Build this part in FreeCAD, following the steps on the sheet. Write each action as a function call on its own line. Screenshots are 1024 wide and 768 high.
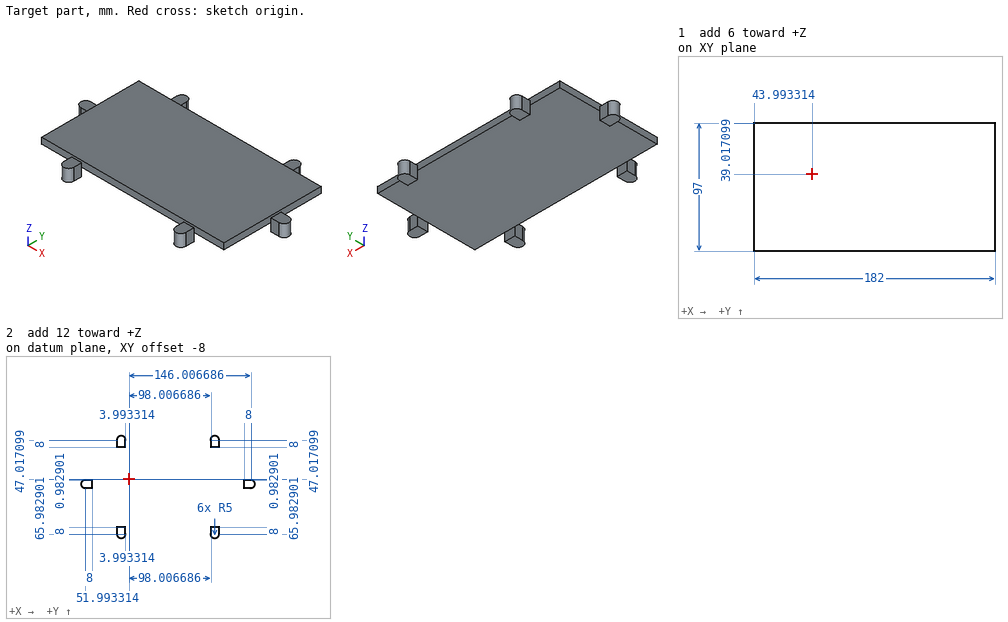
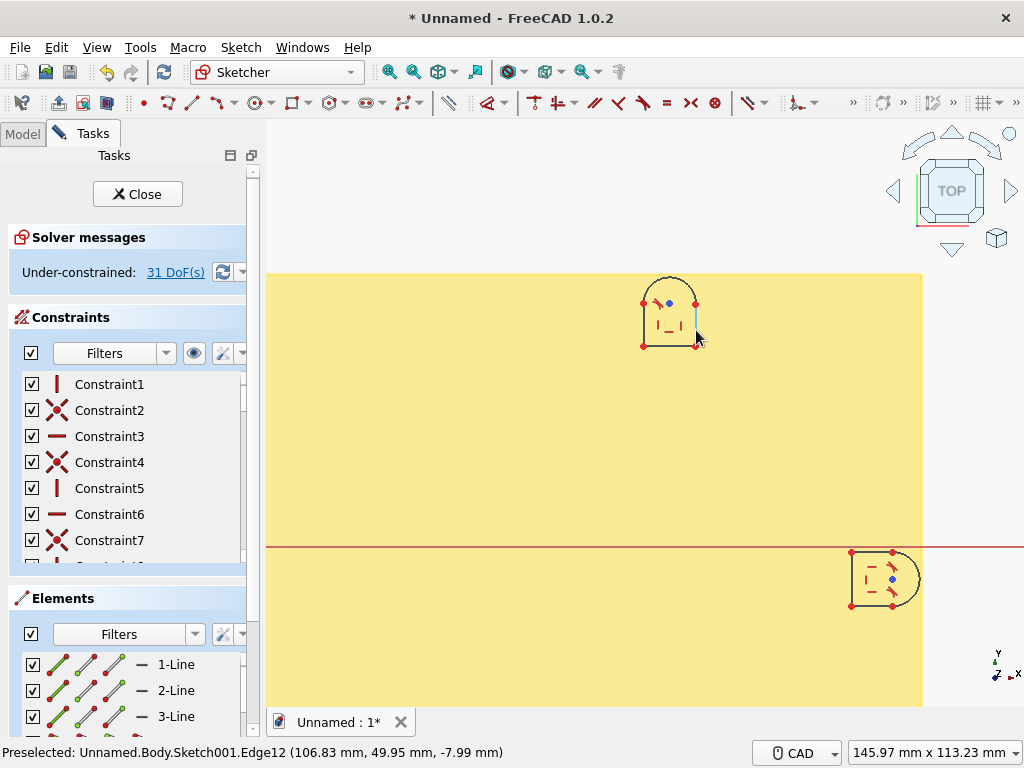
click(696, 329)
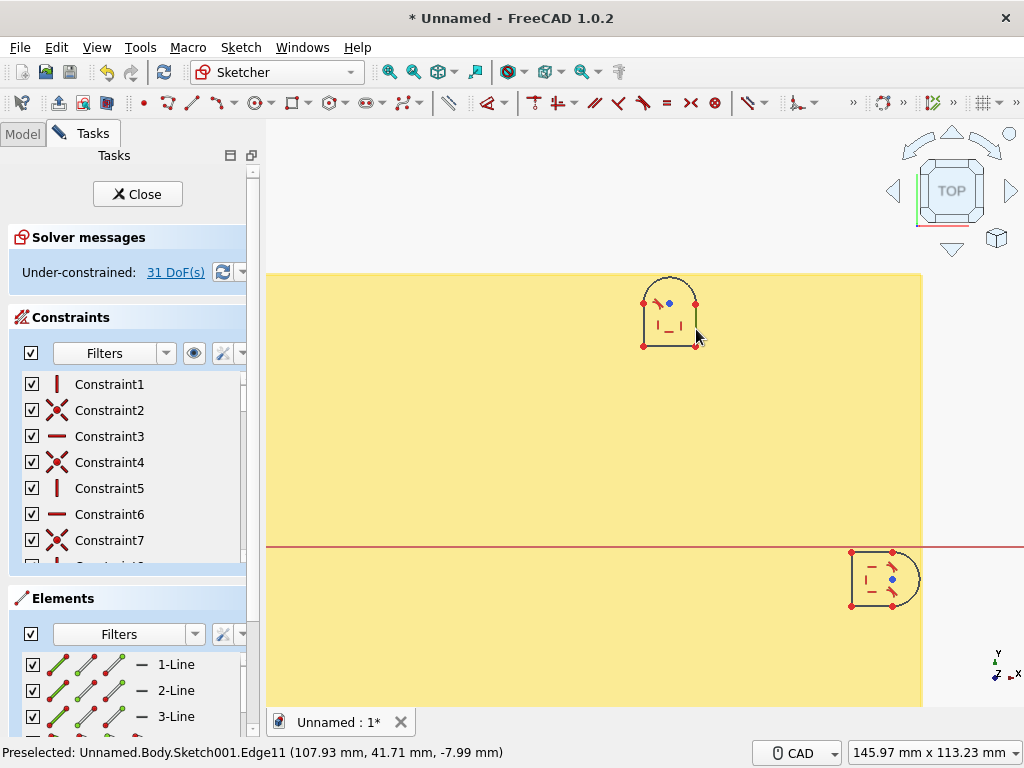
click(685, 283)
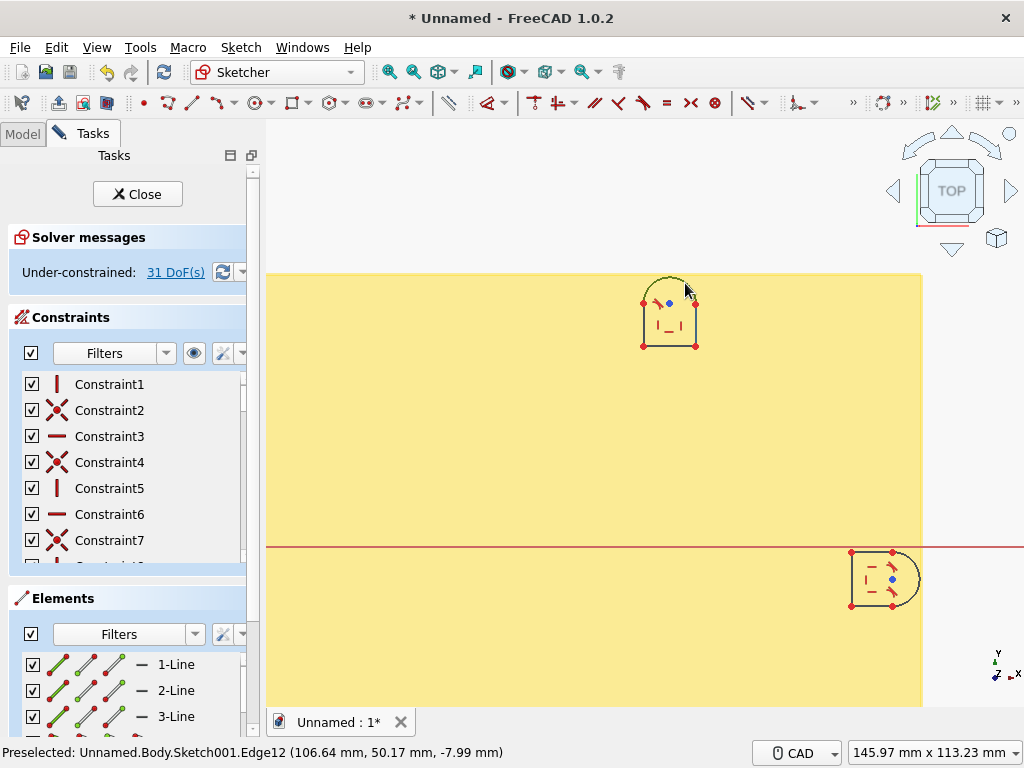
click(644, 104)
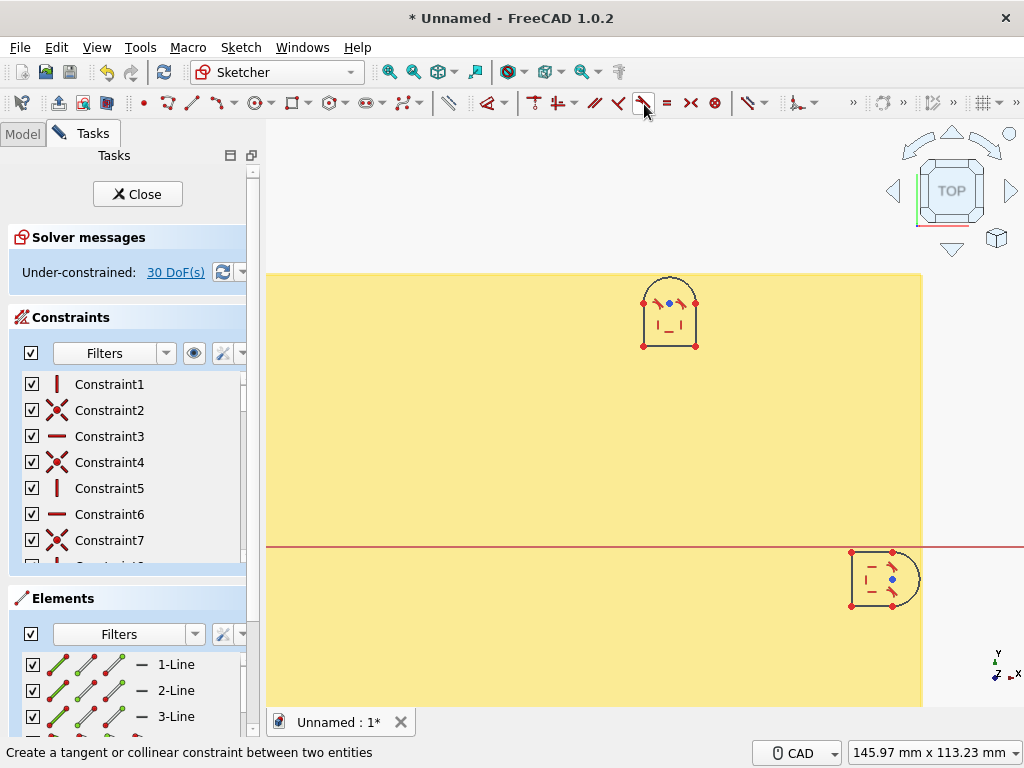
scroll(691, 307, down, 5)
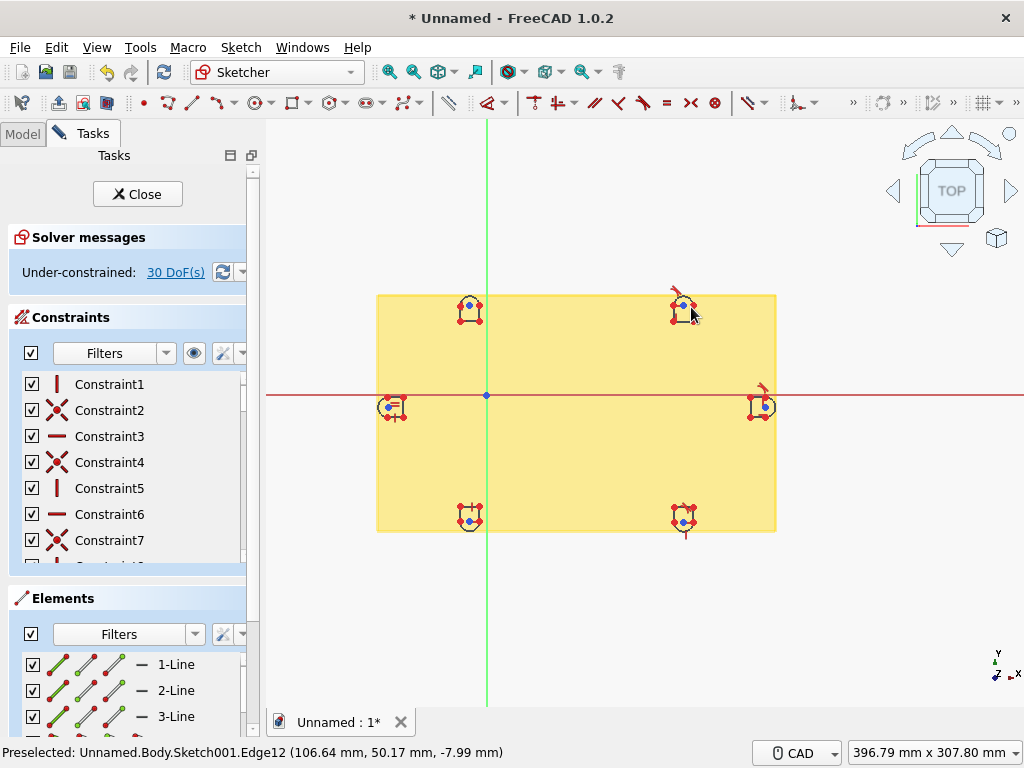
scroll(460, 311, up, 6)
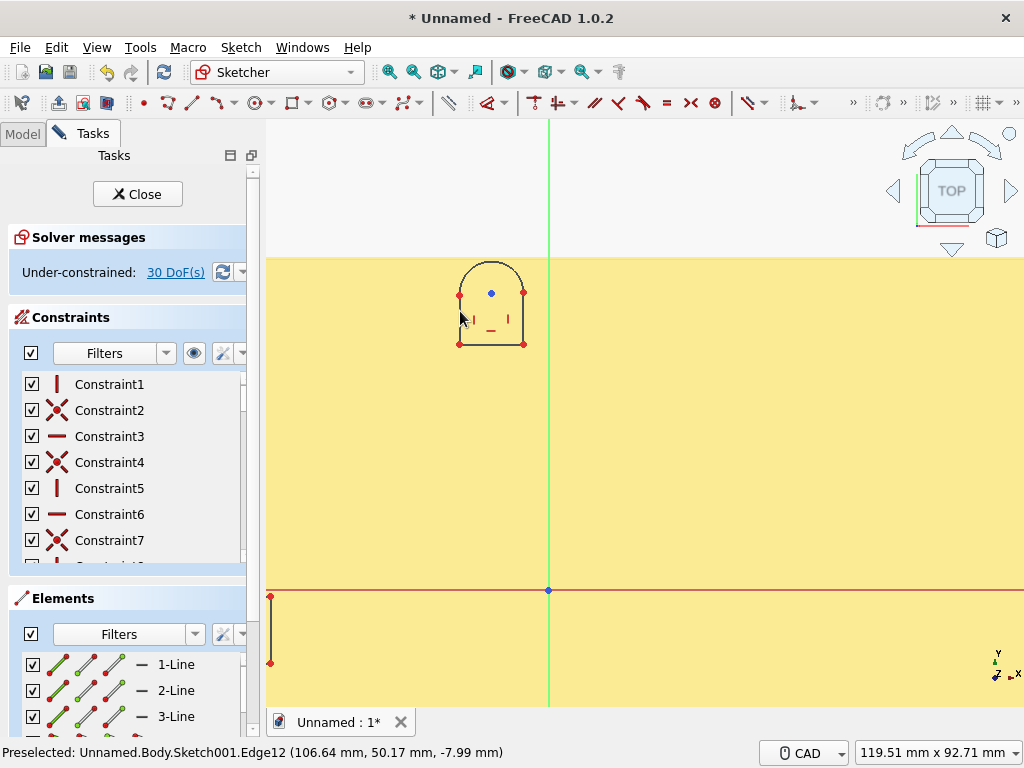
click(460, 310)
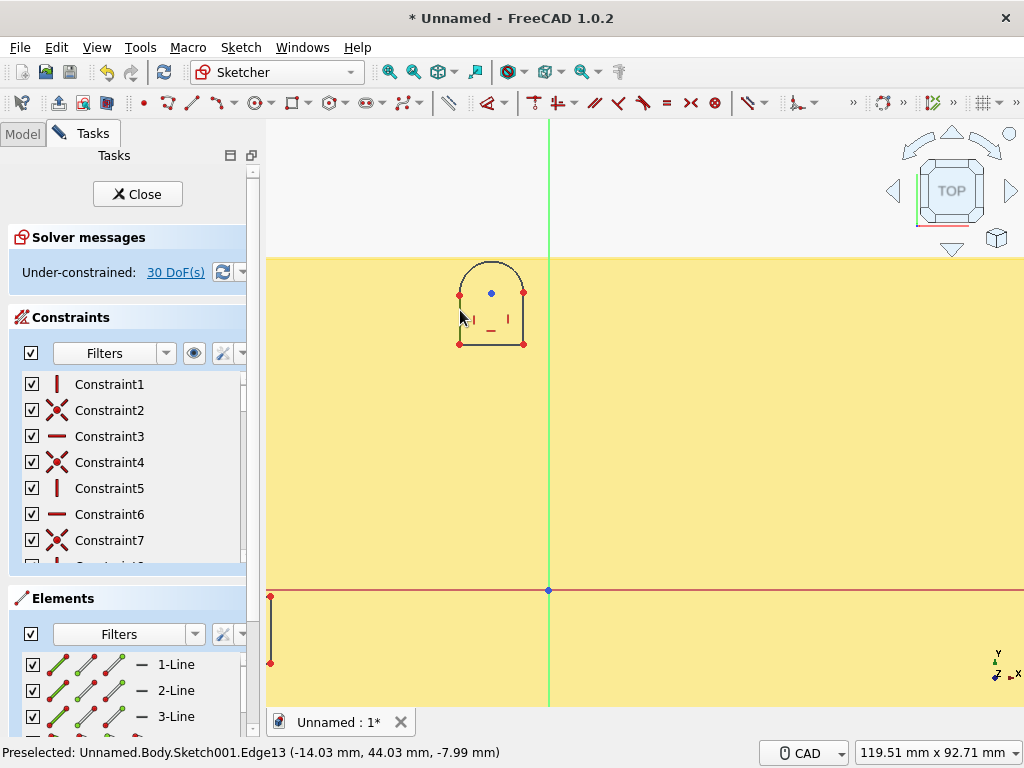
click(510, 267)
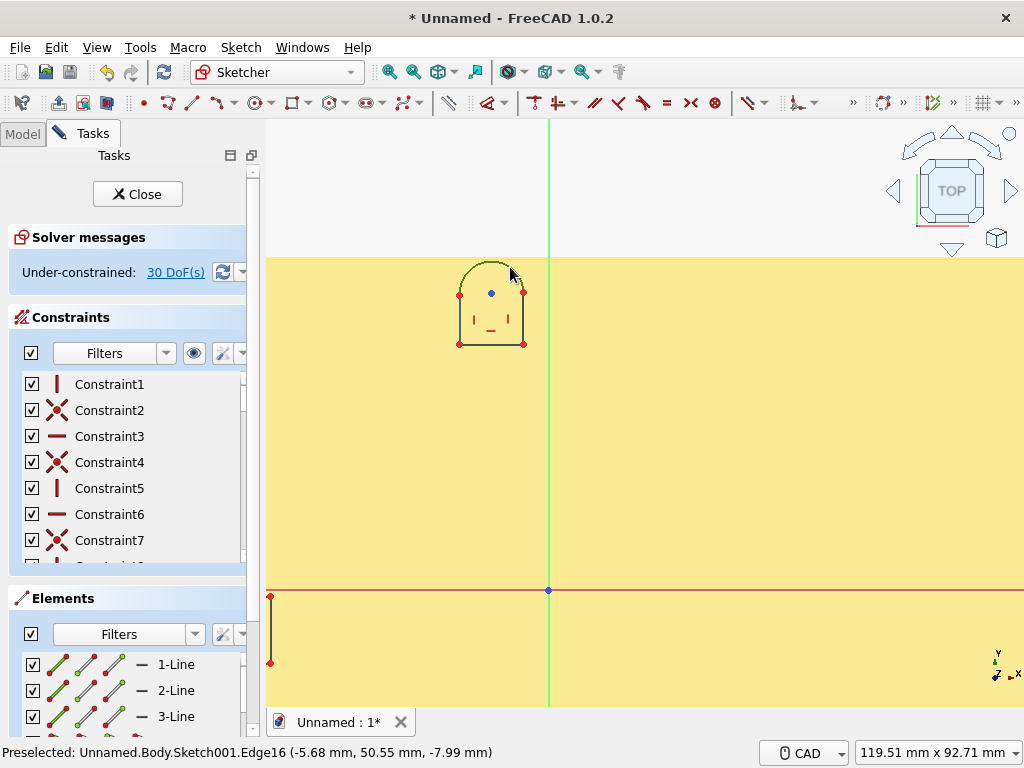
click(644, 104)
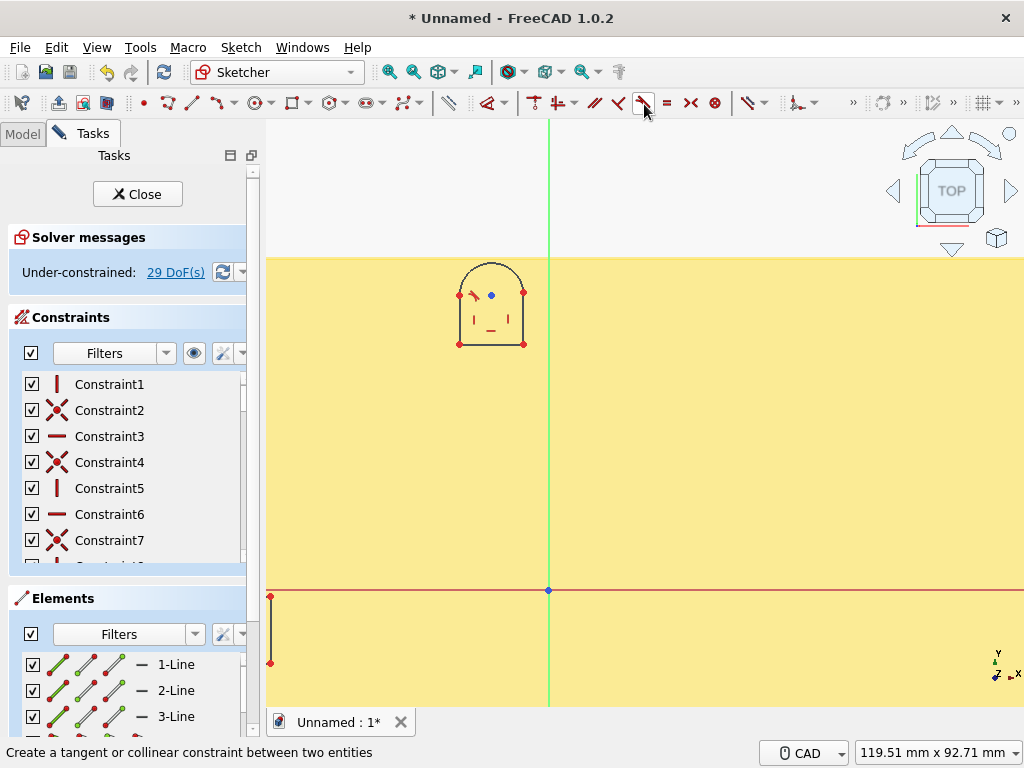
click(524, 329)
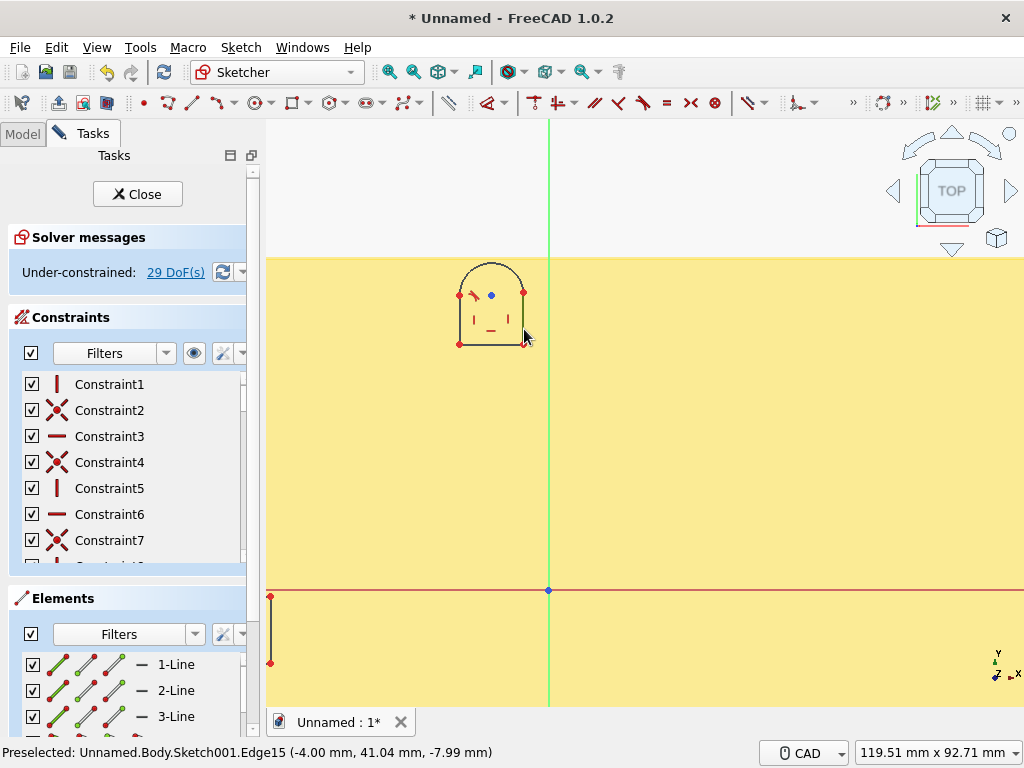
click(509, 268)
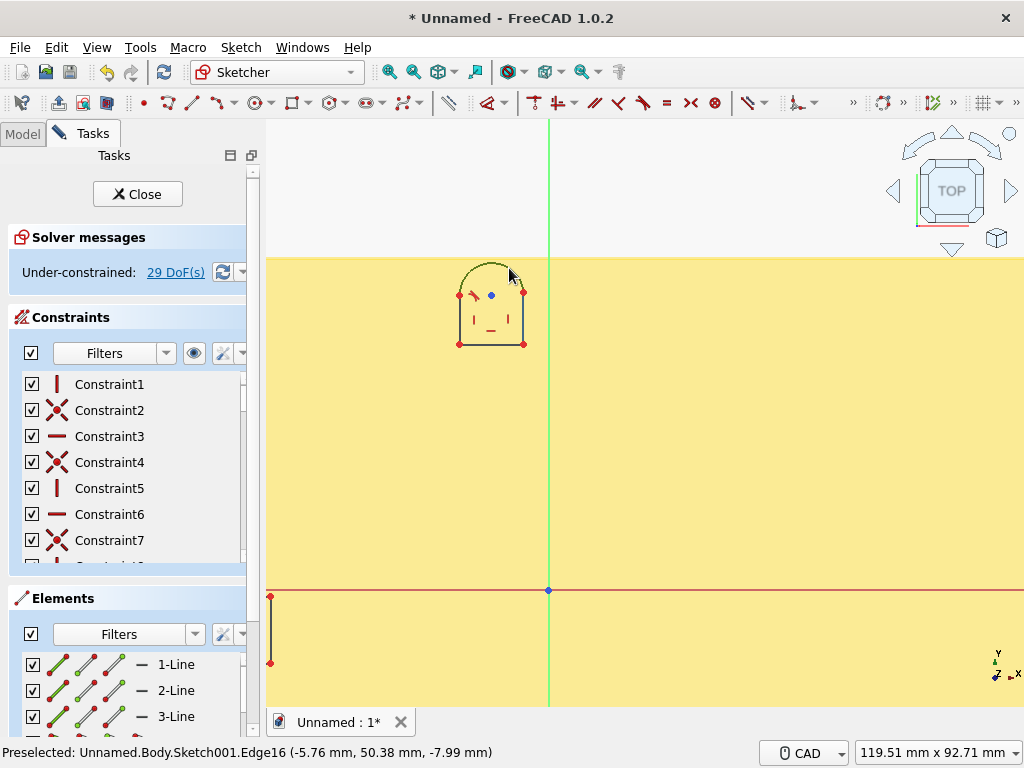
click(644, 104)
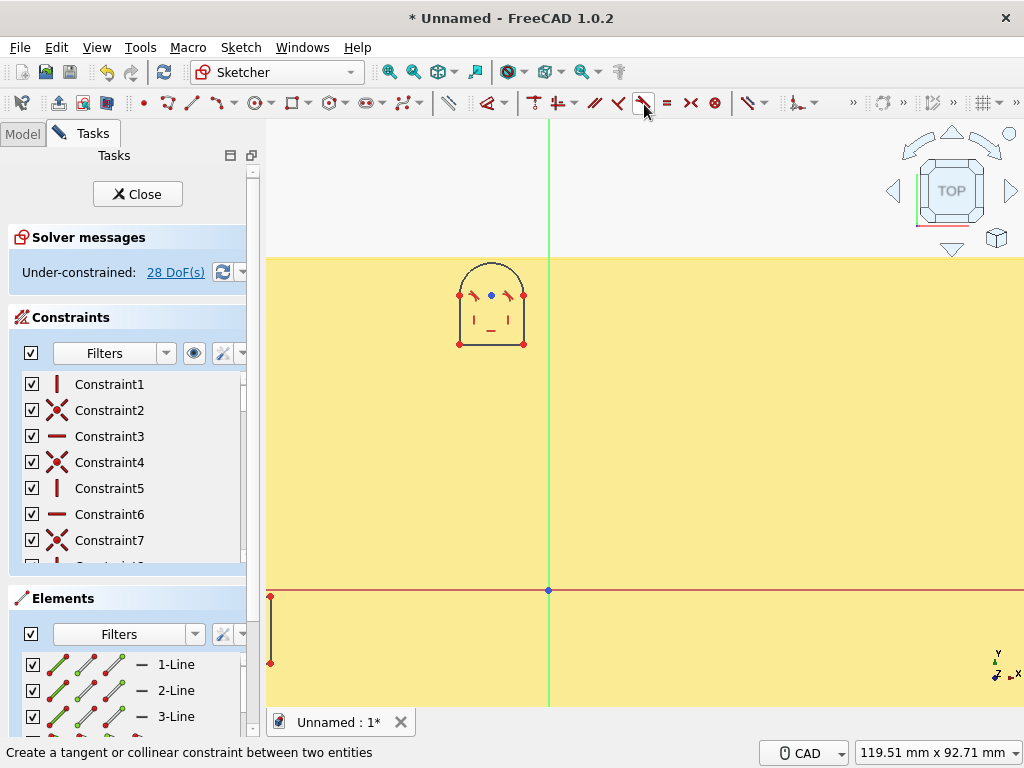
scroll(460, 311, down, 6)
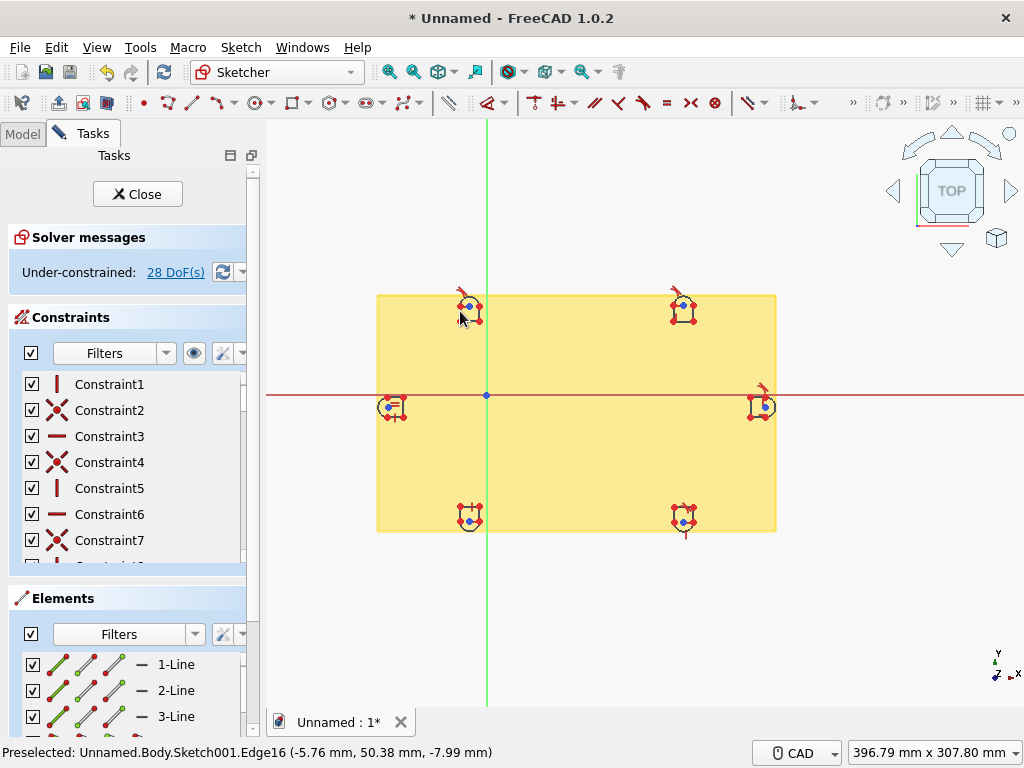
scroll(392, 417, up, 6)